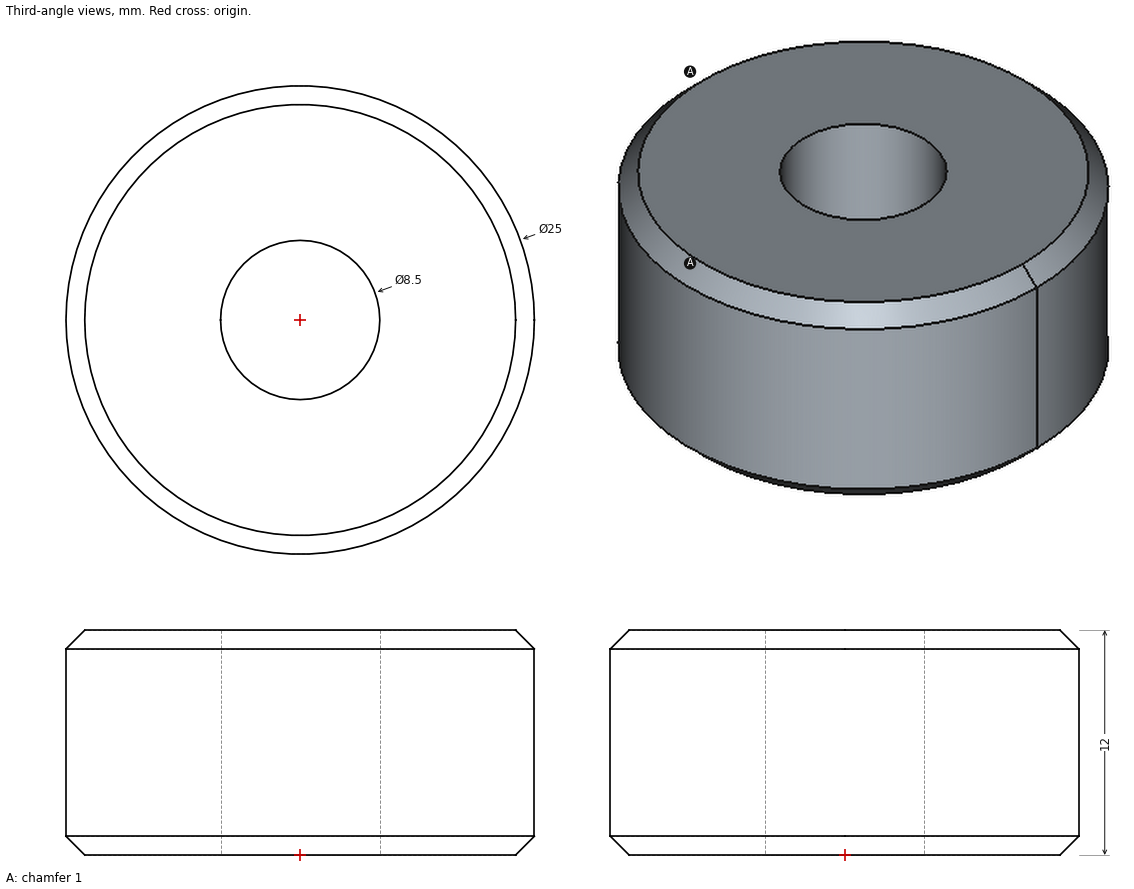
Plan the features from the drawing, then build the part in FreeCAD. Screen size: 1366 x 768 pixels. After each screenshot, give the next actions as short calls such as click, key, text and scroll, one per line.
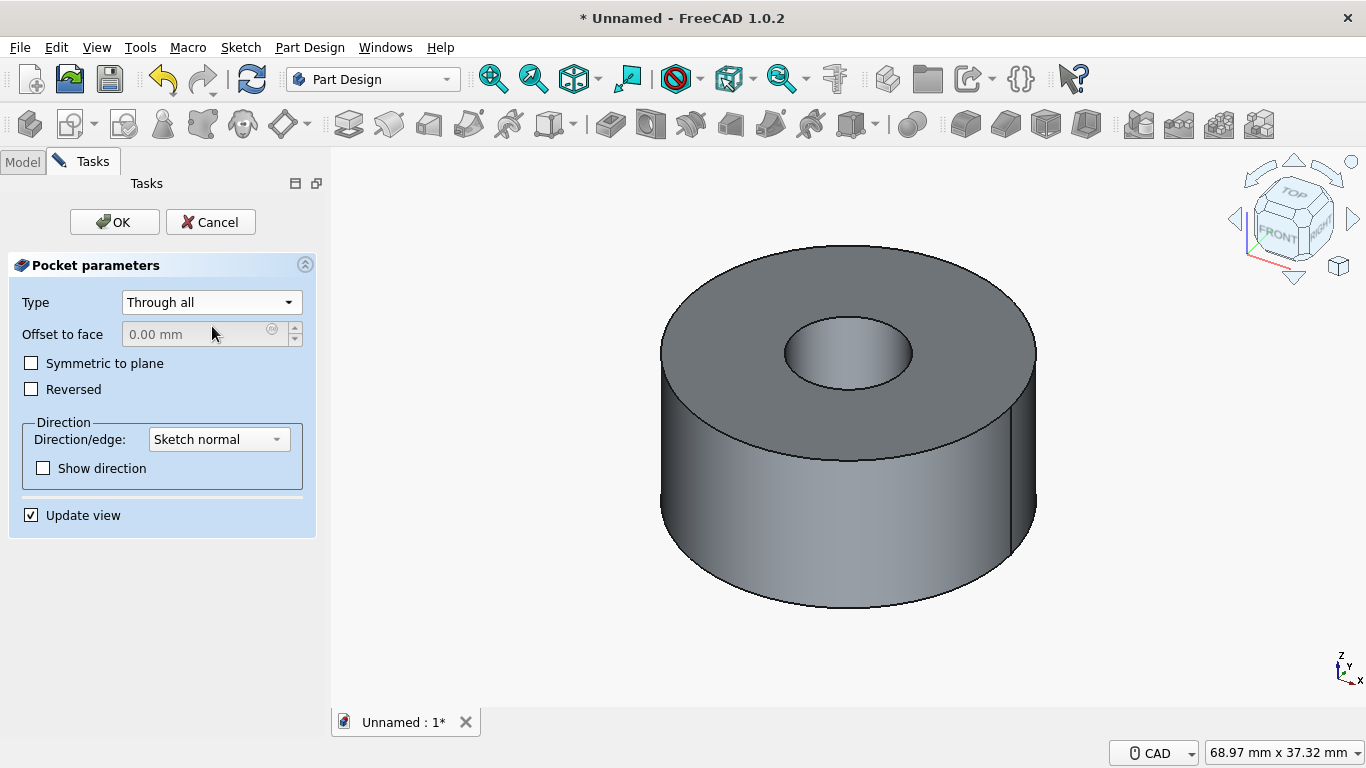
click(115, 222)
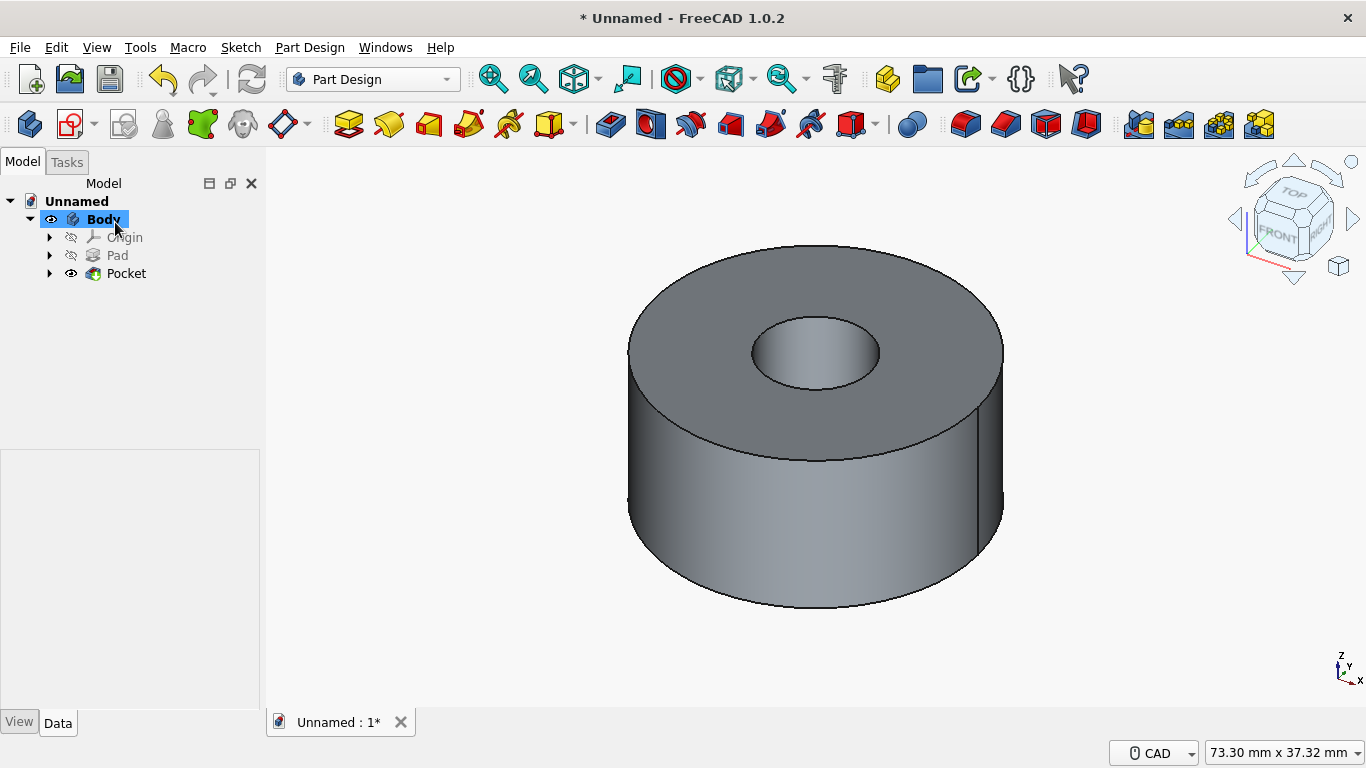
click(629, 363)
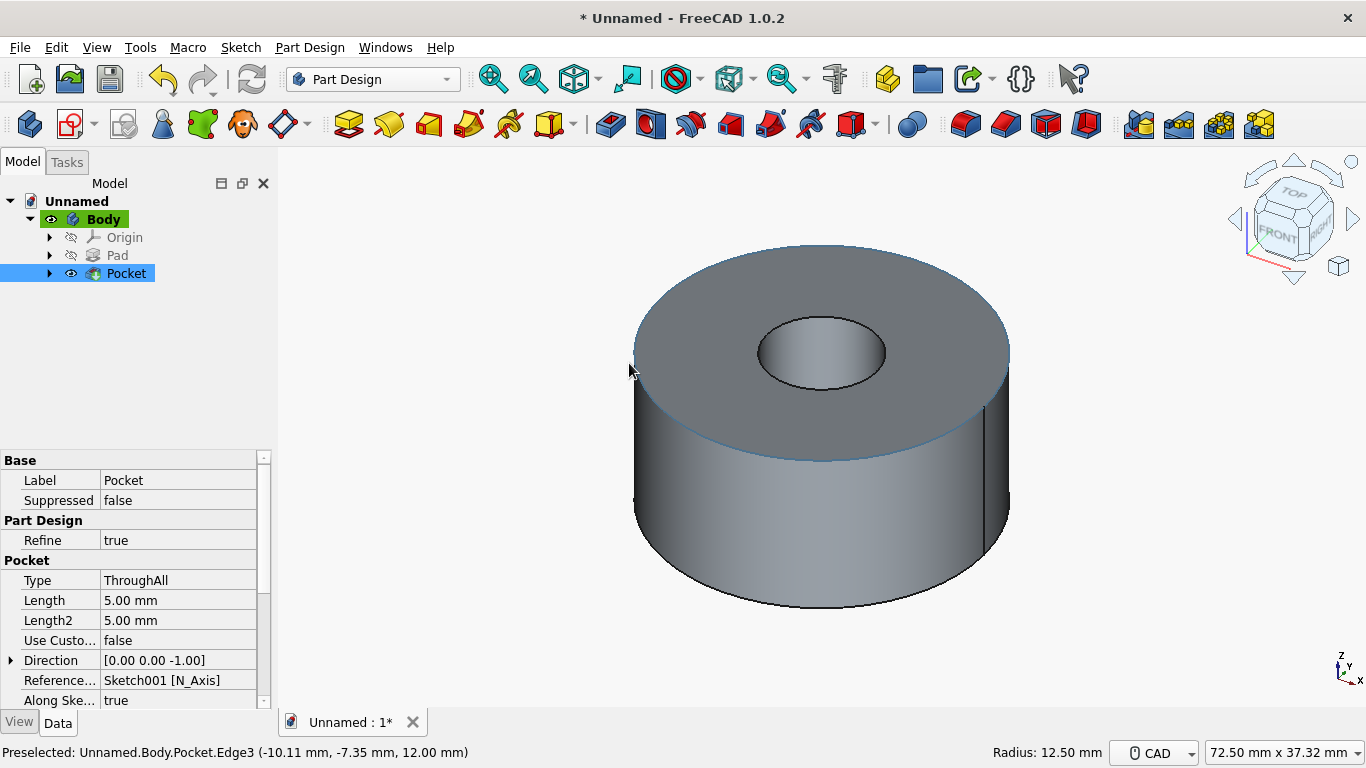
key(0)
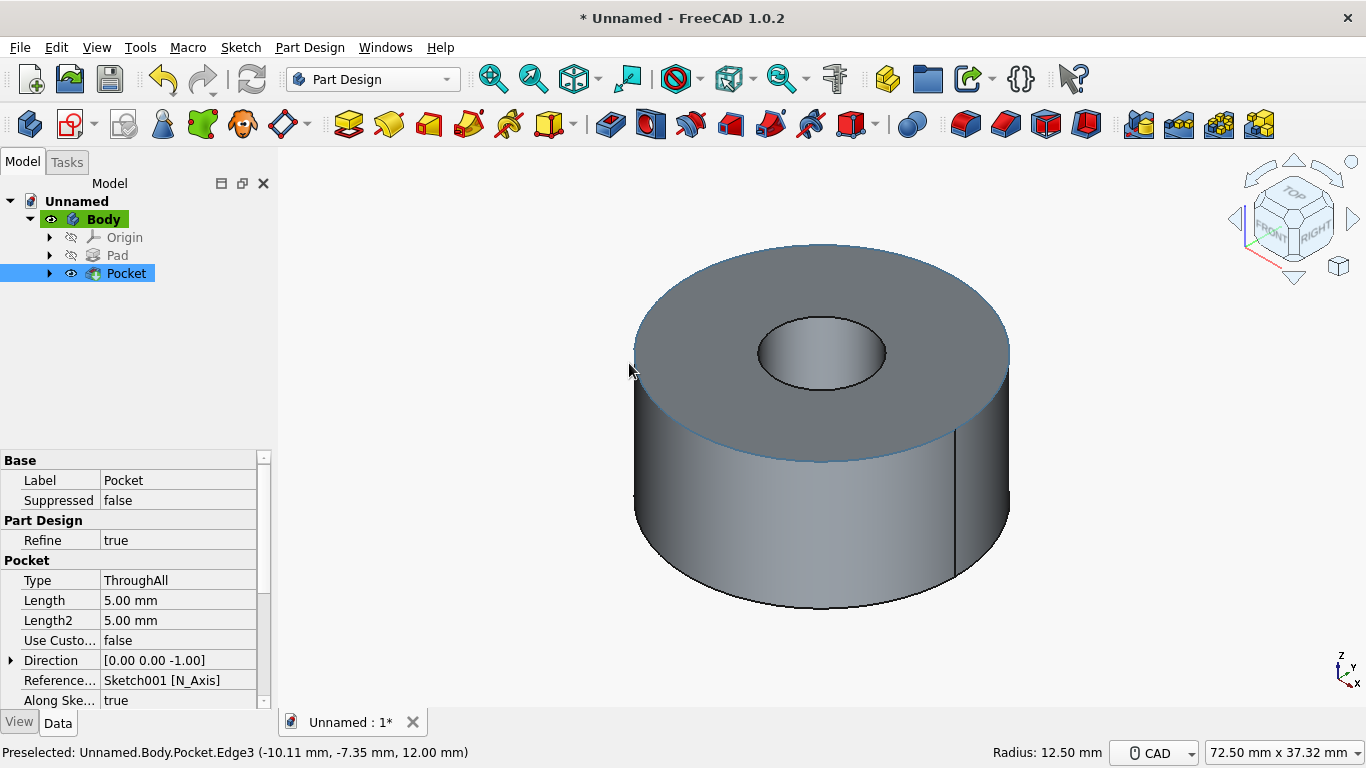
key(2)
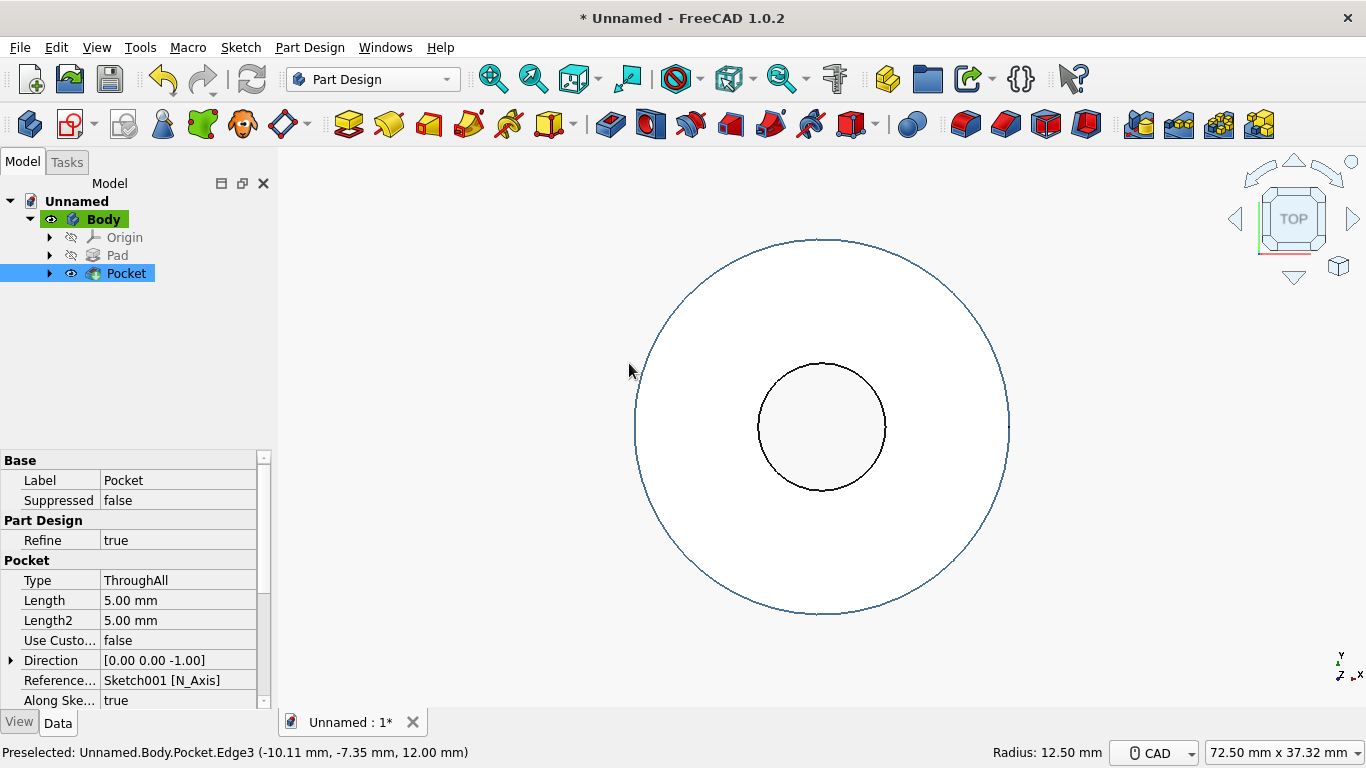
key(1)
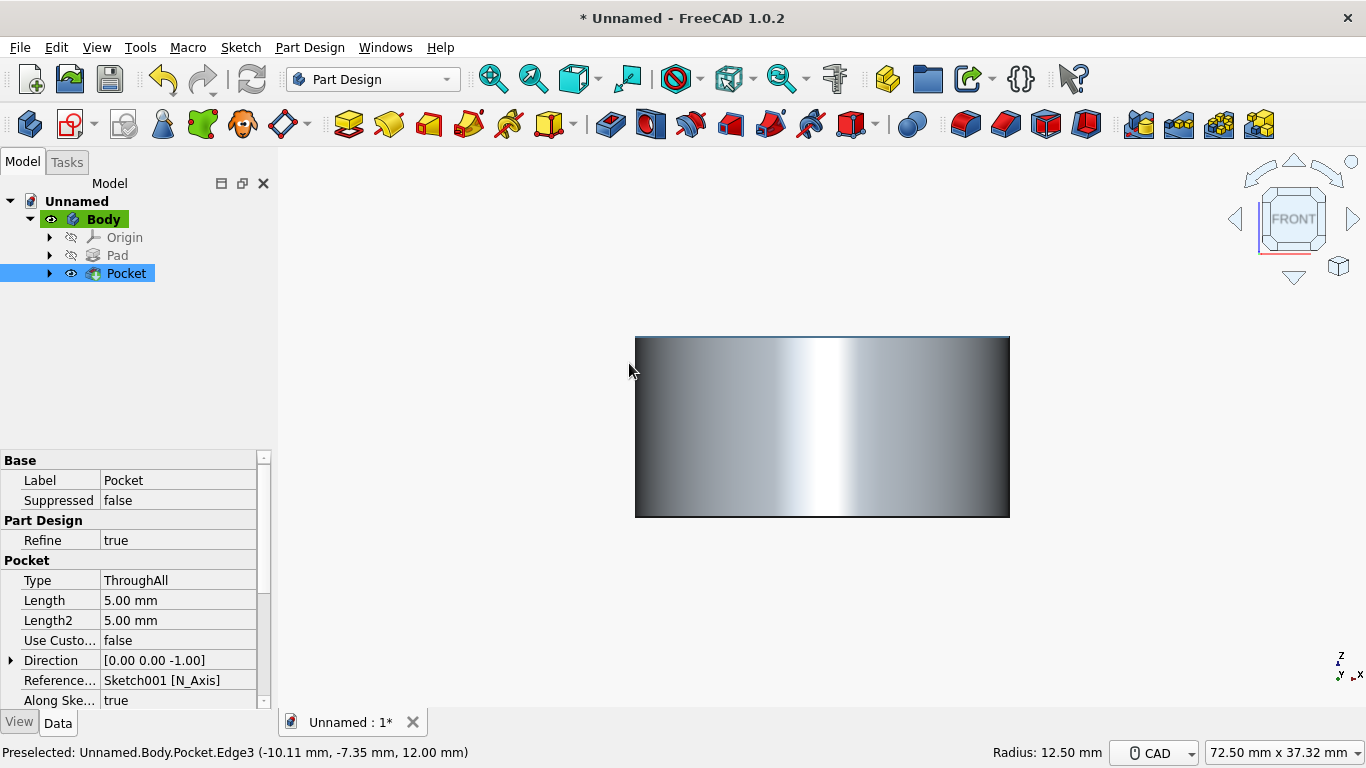
key(v)
key(f)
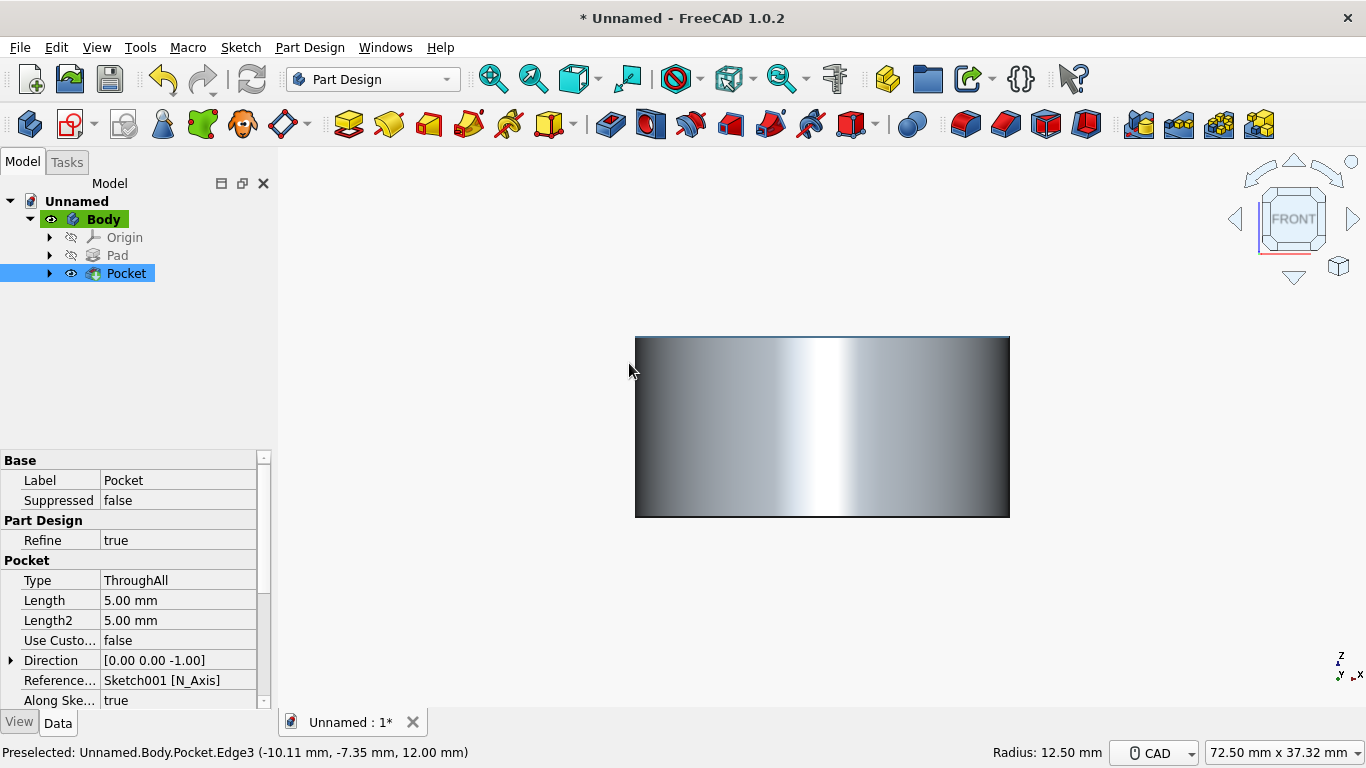
click(670, 516, ctrl)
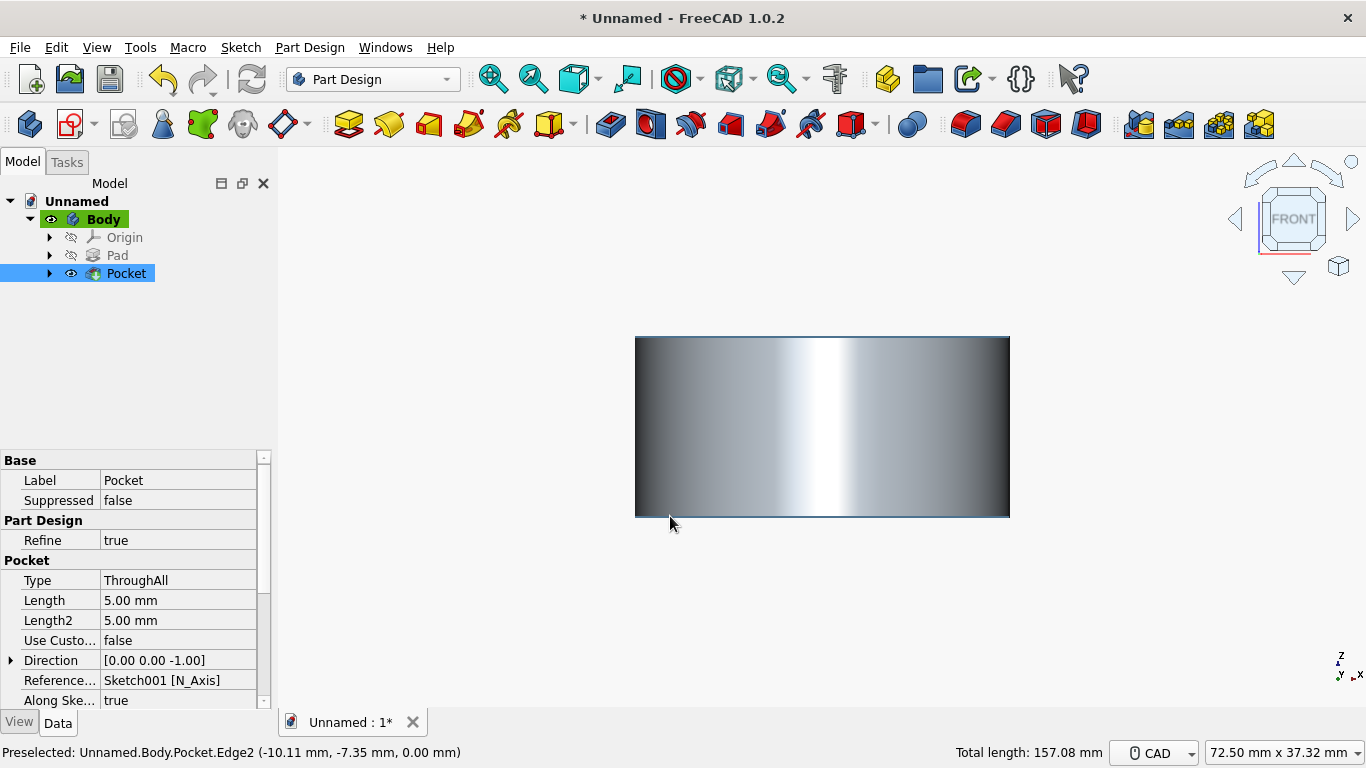
click(1006, 124)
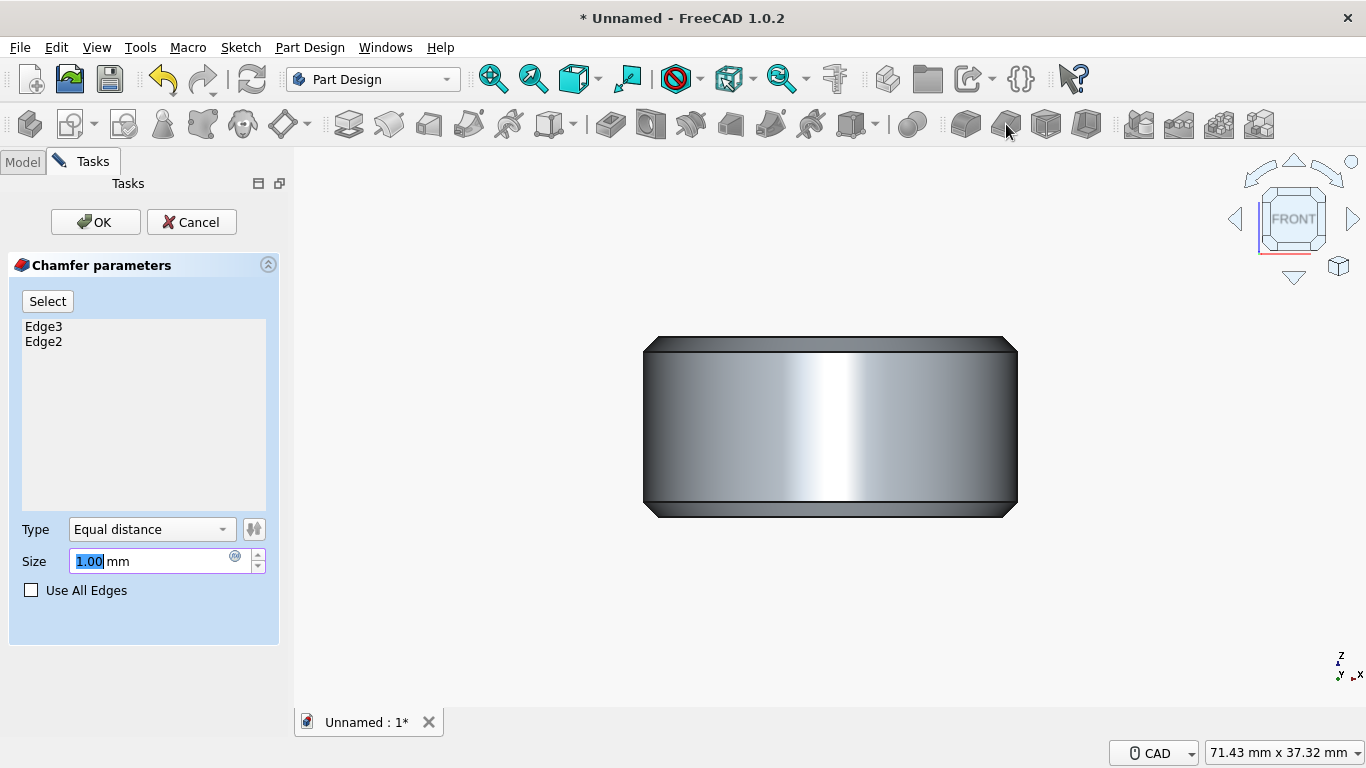
text(1)
key(Tab)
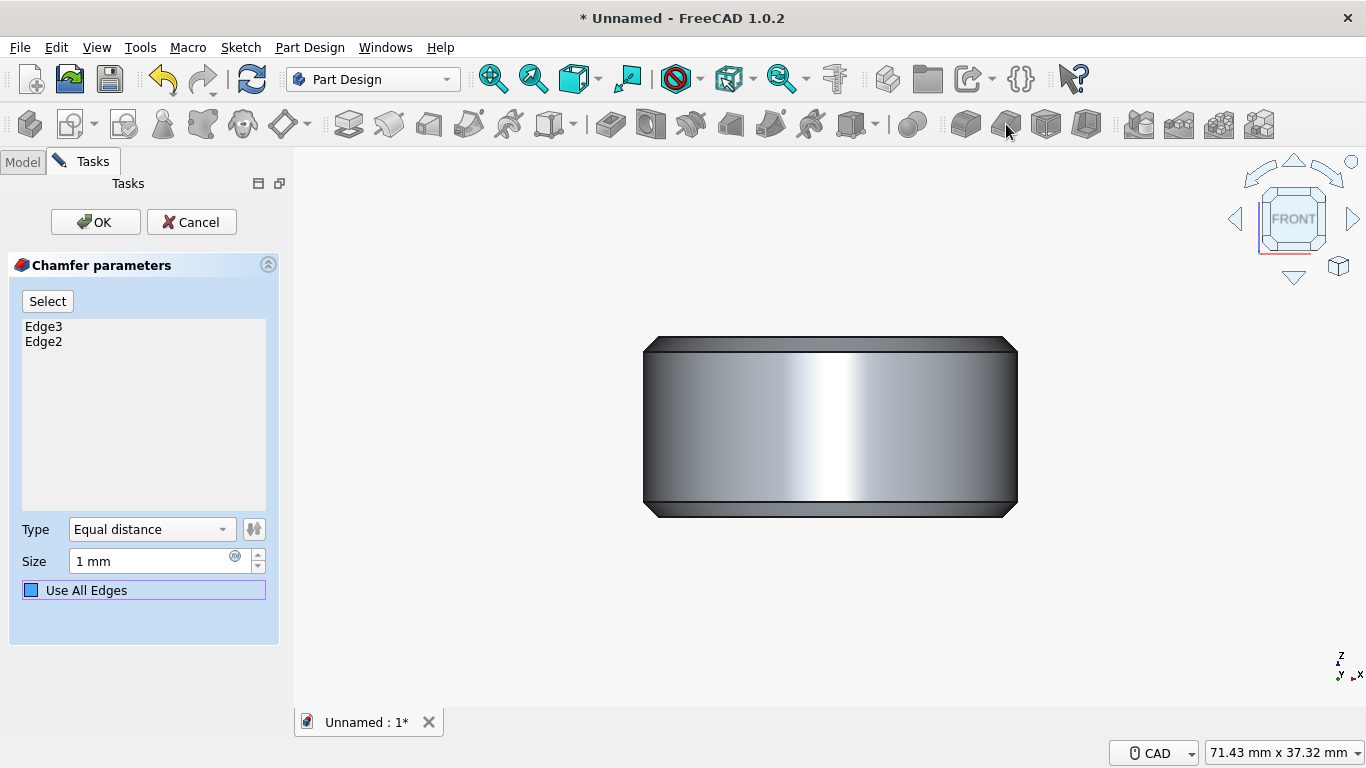
click(96, 222)